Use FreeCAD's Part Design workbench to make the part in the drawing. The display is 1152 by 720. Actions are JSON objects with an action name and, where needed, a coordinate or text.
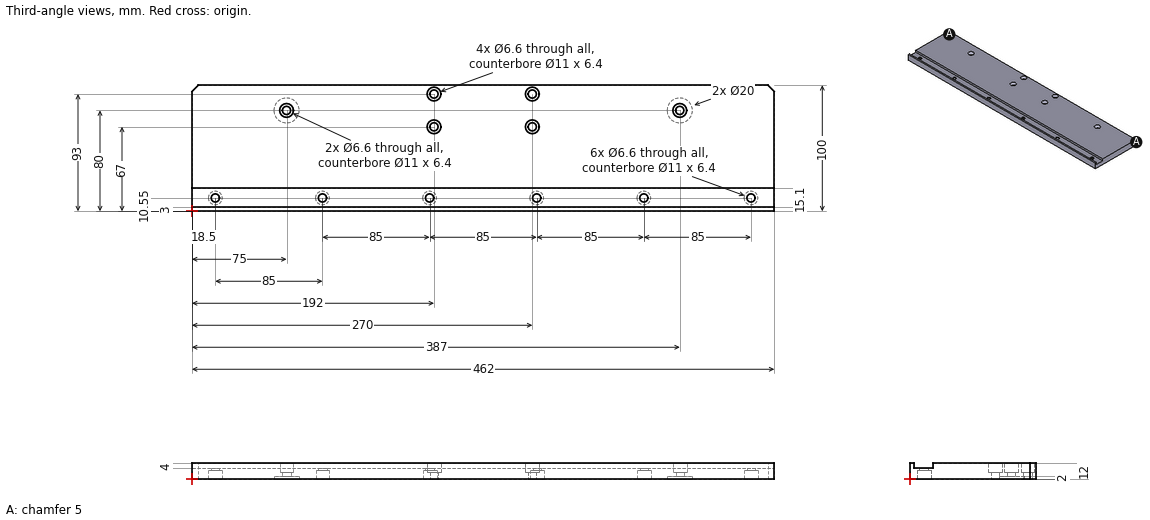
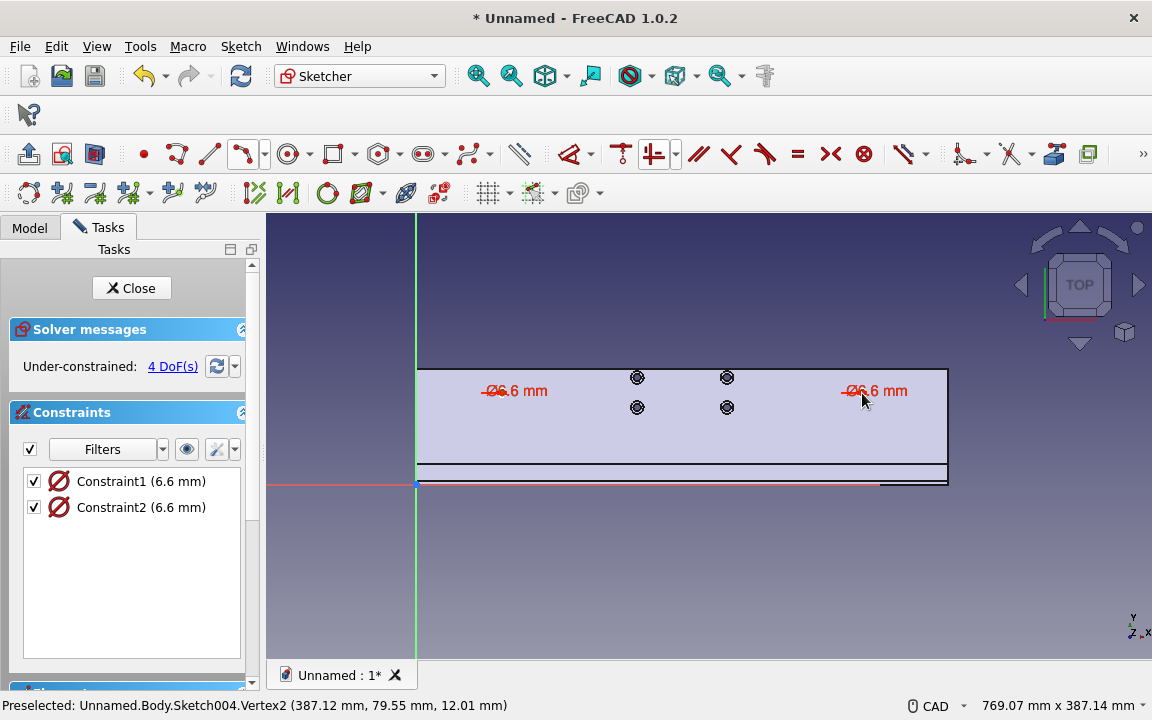
{"action": "left_click", "coordinate": [676, 154]}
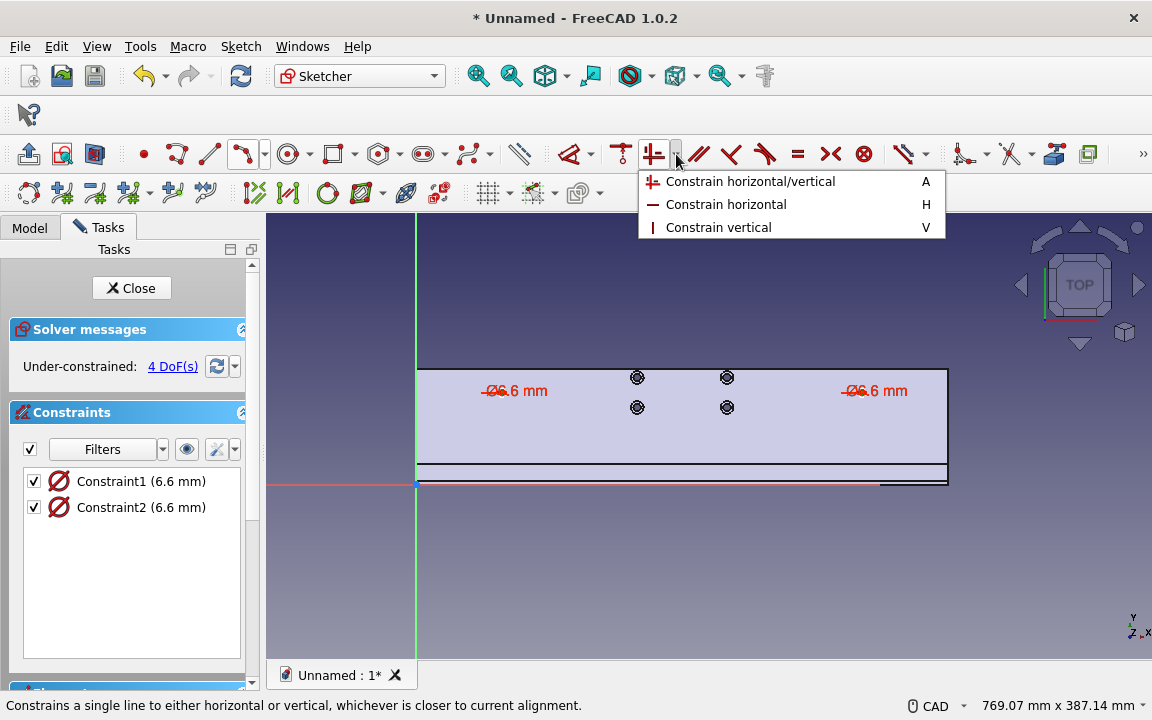
{"action": "left_click", "coordinate": [792, 204]}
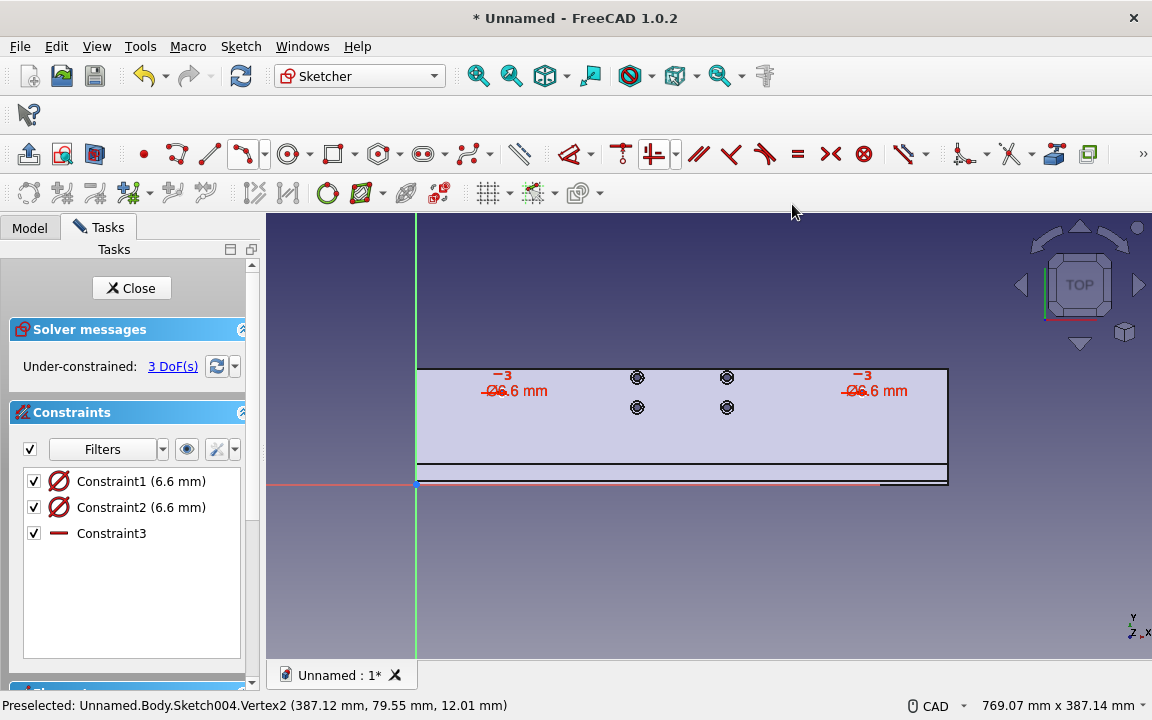
{"action": "left_click", "coordinate": [568, 154]}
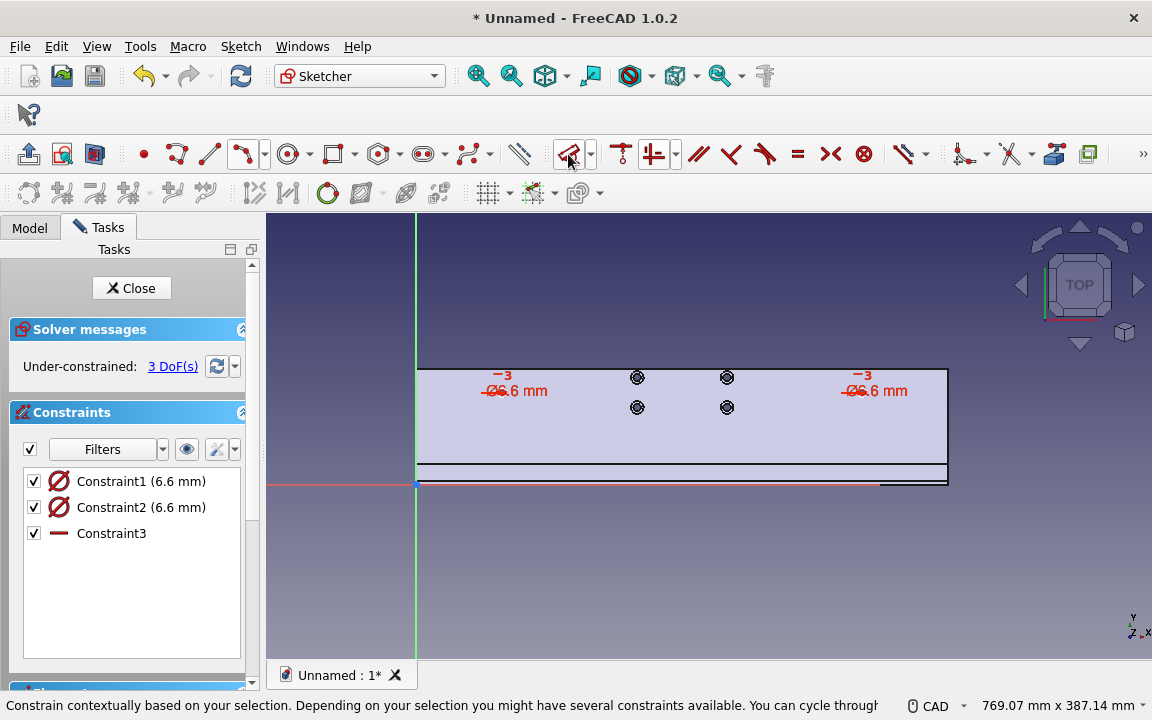
{"action": "left_click", "coordinate": [502, 393]}
{"action": "left_click", "coordinate": [459, 519]}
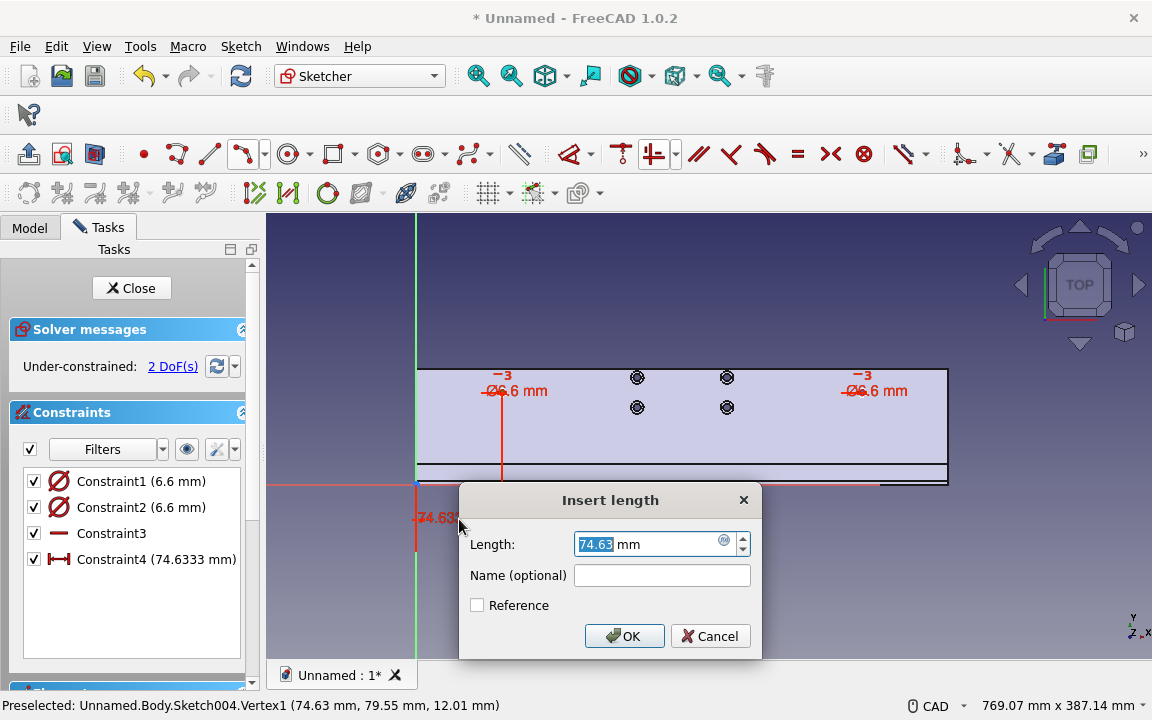
{"action": "type", "text": "75"}
{"action": "key", "text": "Return"}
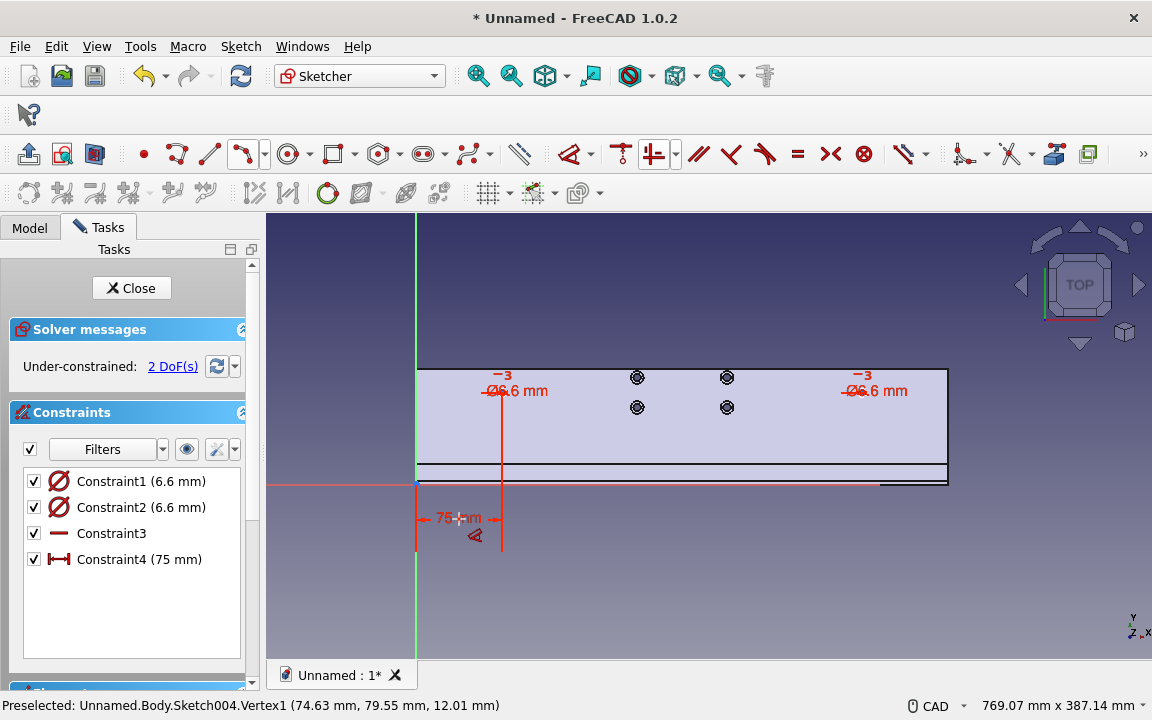
{"action": "left_click", "coordinate": [502, 393]}
{"action": "left_click", "coordinate": [382, 439]}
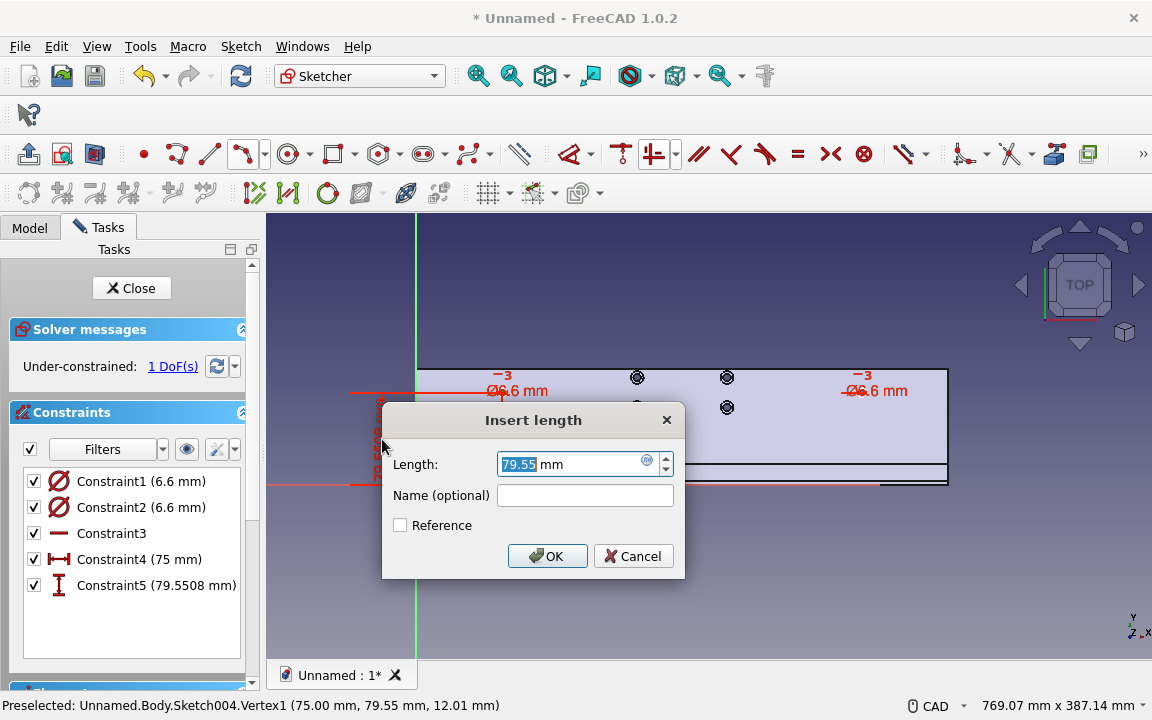
{"action": "type", "text": "80"}
{"action": "key", "text": "Return"}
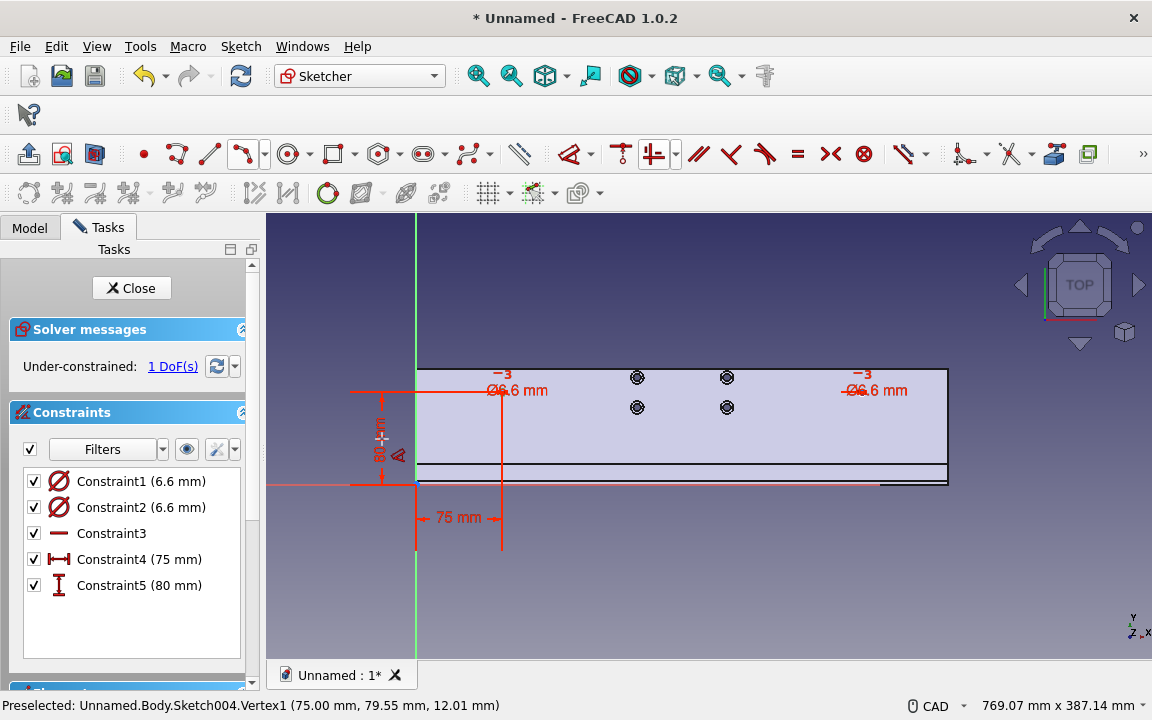
{"action": "left_click", "coordinate": [862, 392]}
{"action": "left_click", "coordinate": [639, 519]}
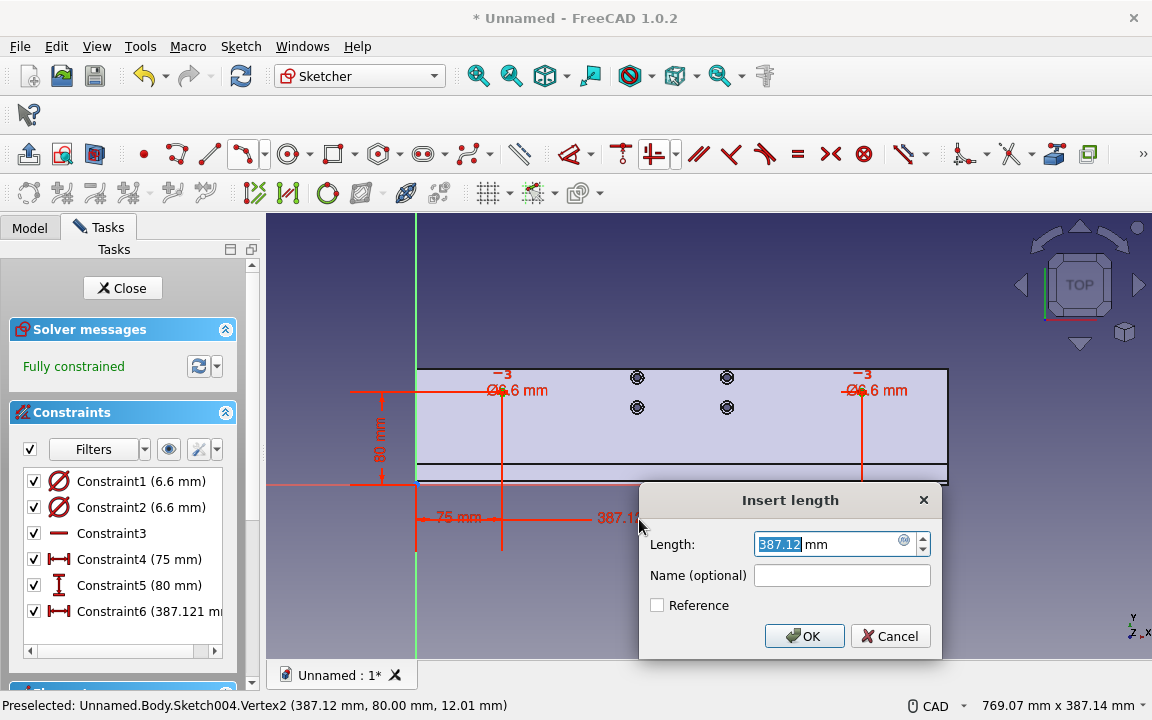
{"action": "type", "text": "387"}
{"action": "key", "text": "Return"}
{"action": "key", "text": "Escape"}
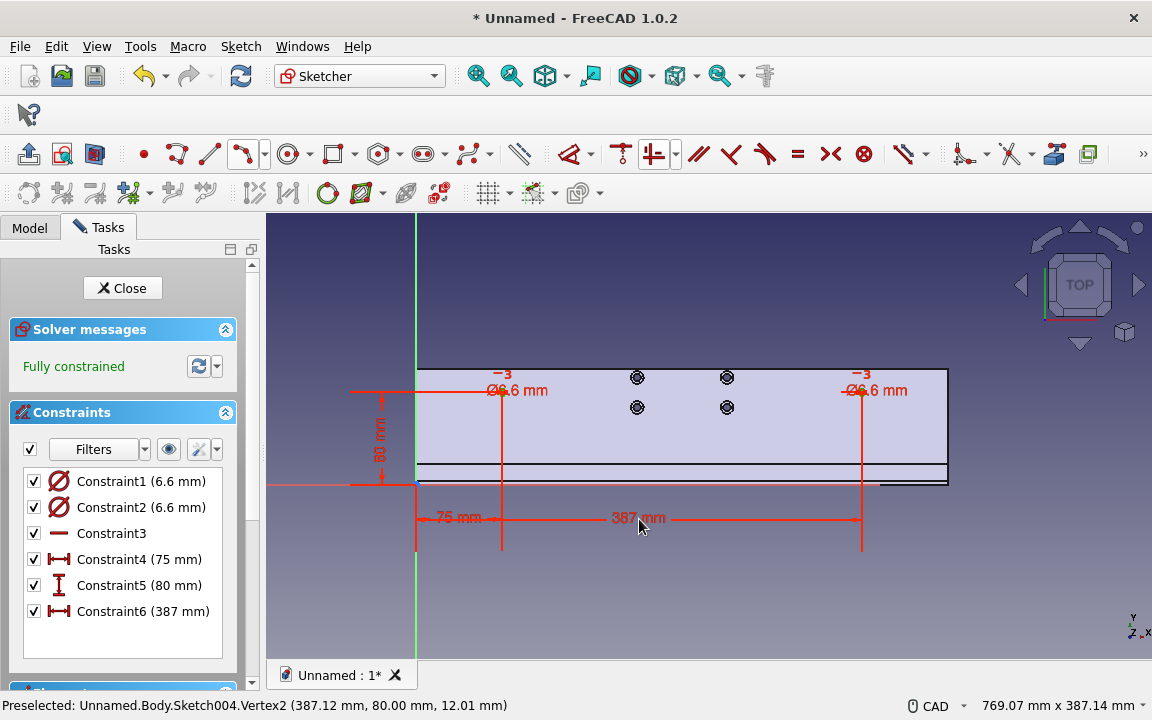
{"action": "left_click", "coordinate": [123, 288]}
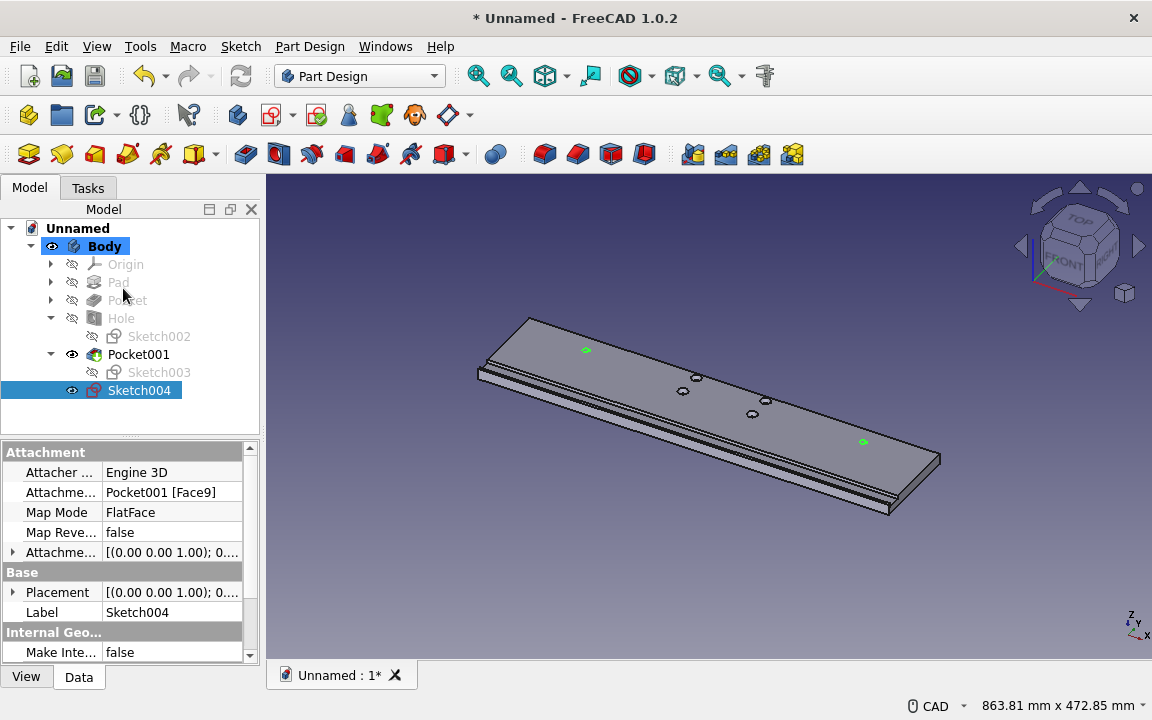
{"action": "left_click", "coordinate": [279, 154]}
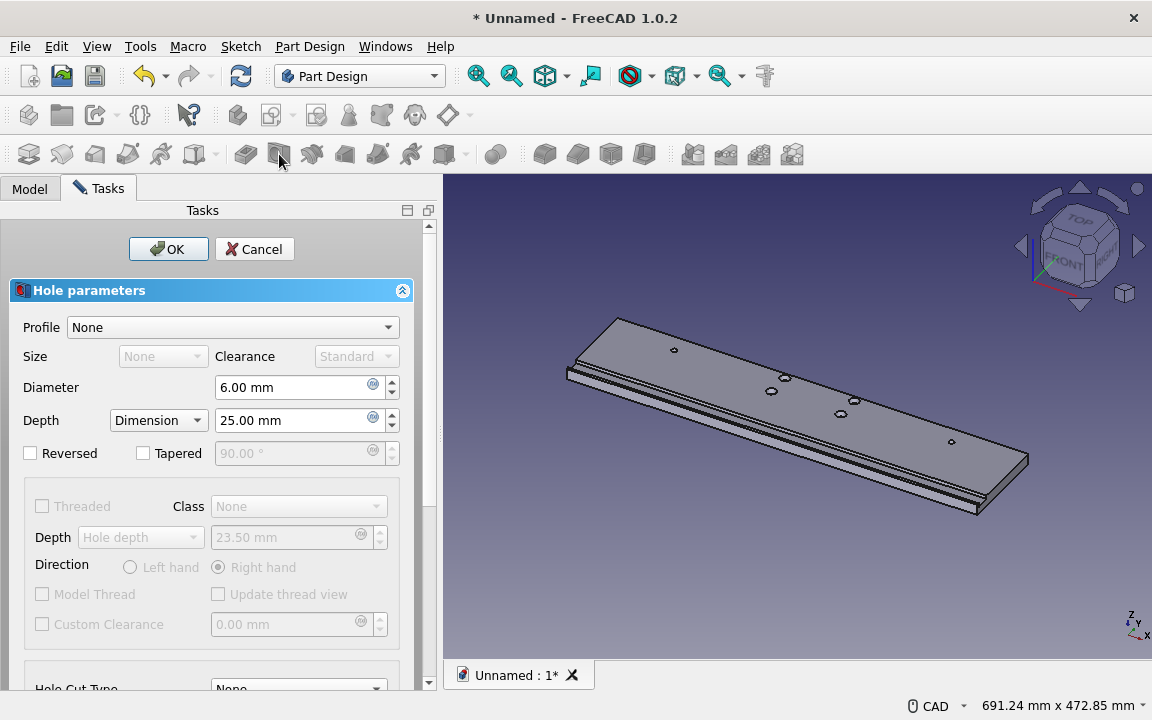
{"action": "triple_click", "coordinate": [300, 388]}